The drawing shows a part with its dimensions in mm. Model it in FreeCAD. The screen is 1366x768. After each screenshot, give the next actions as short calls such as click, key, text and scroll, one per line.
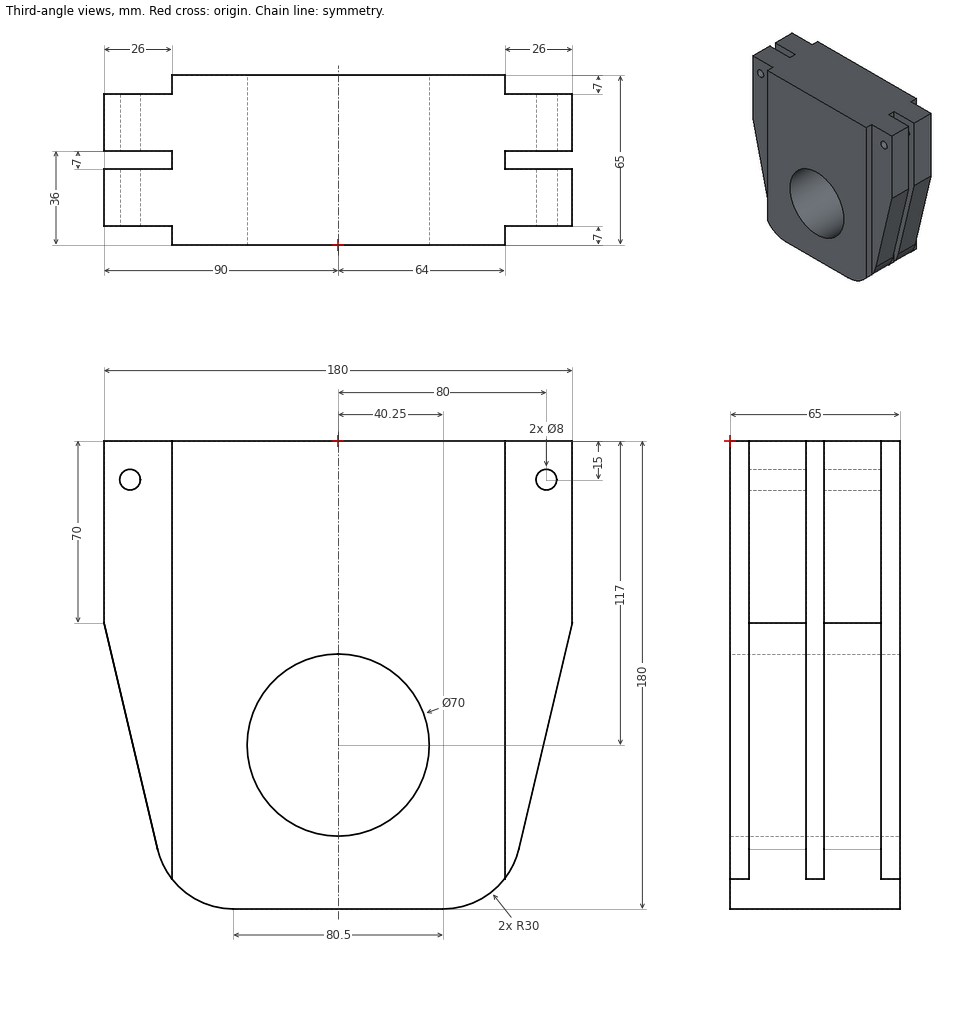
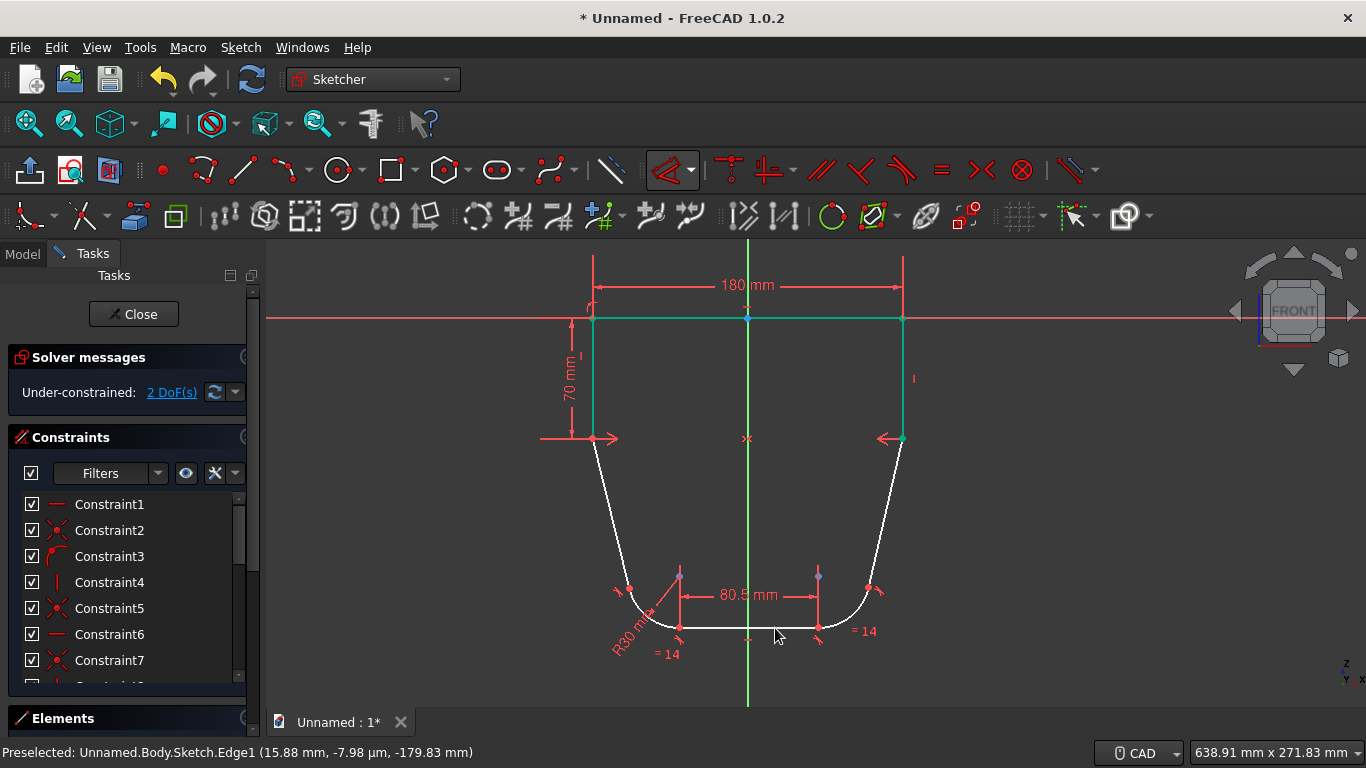
click(818, 628)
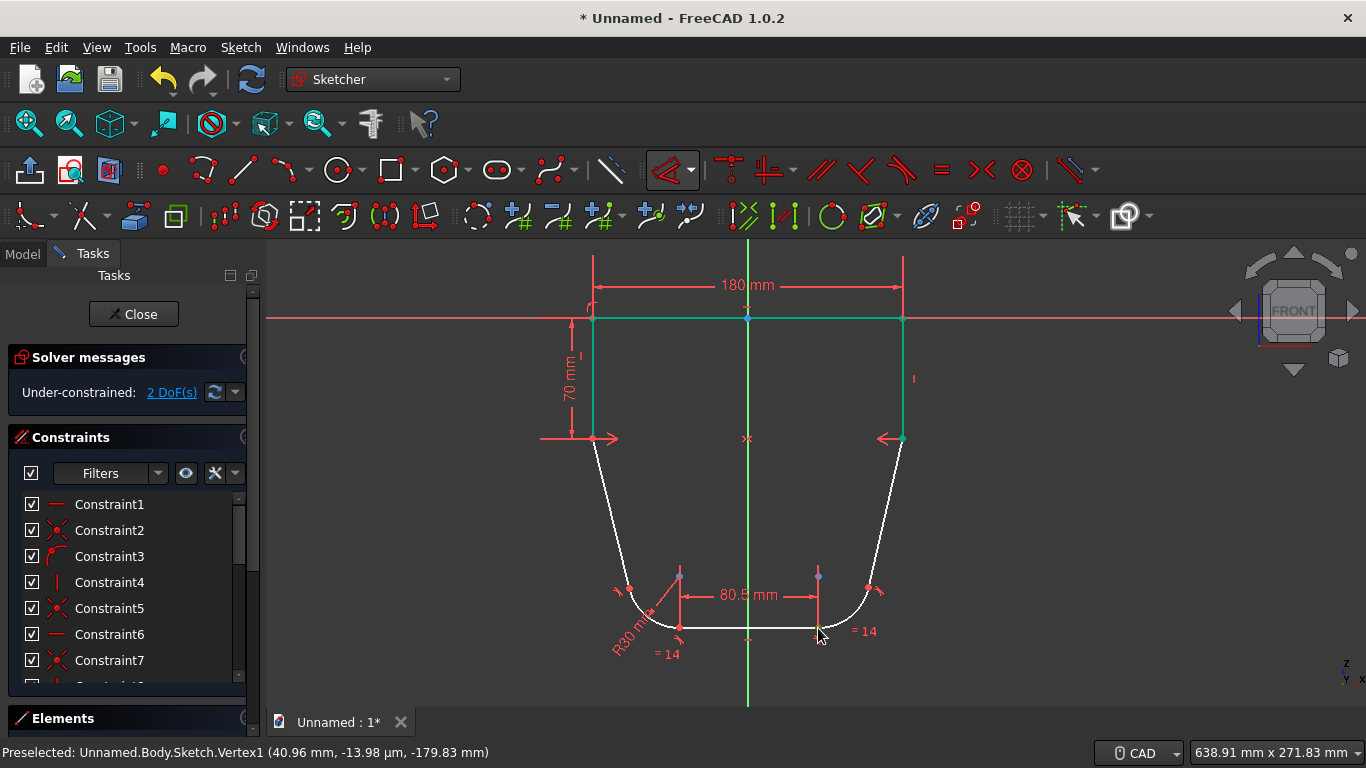
click(694, 170)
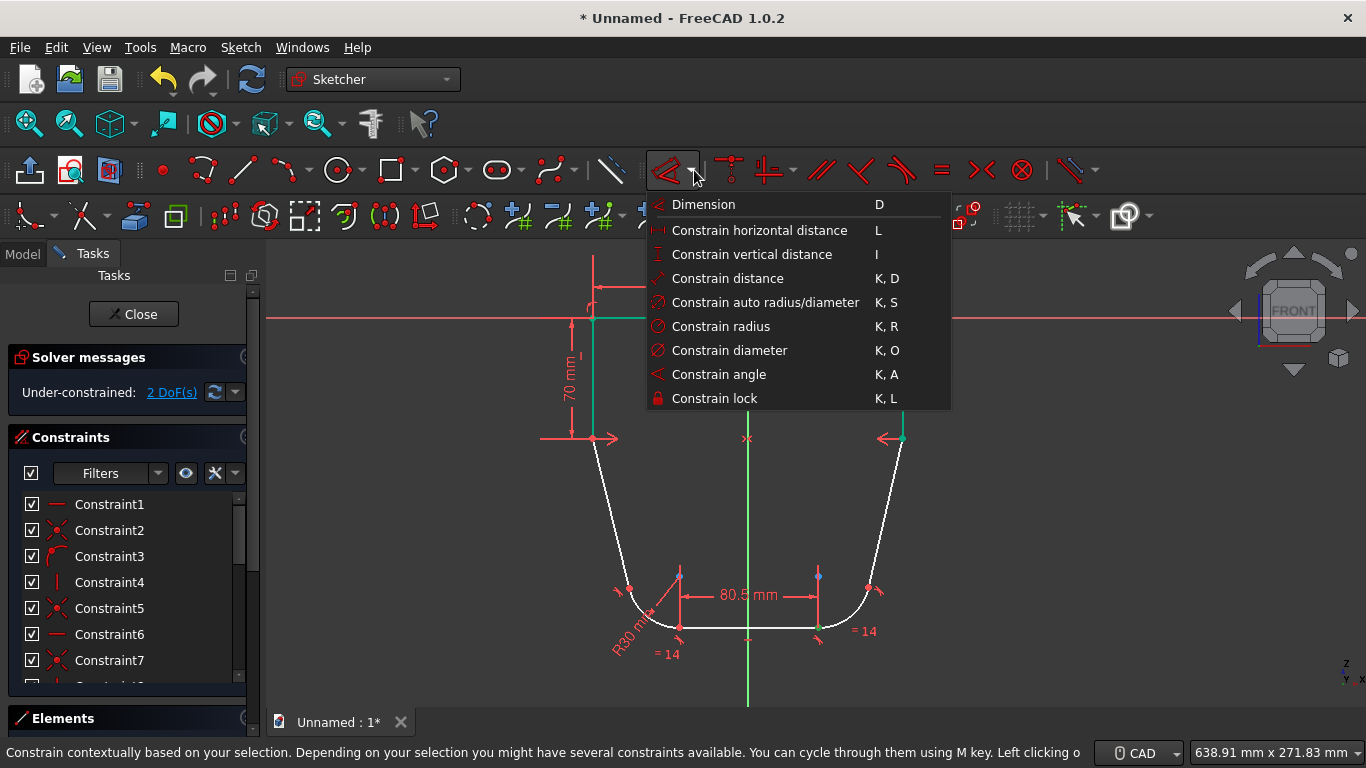
click(799, 254)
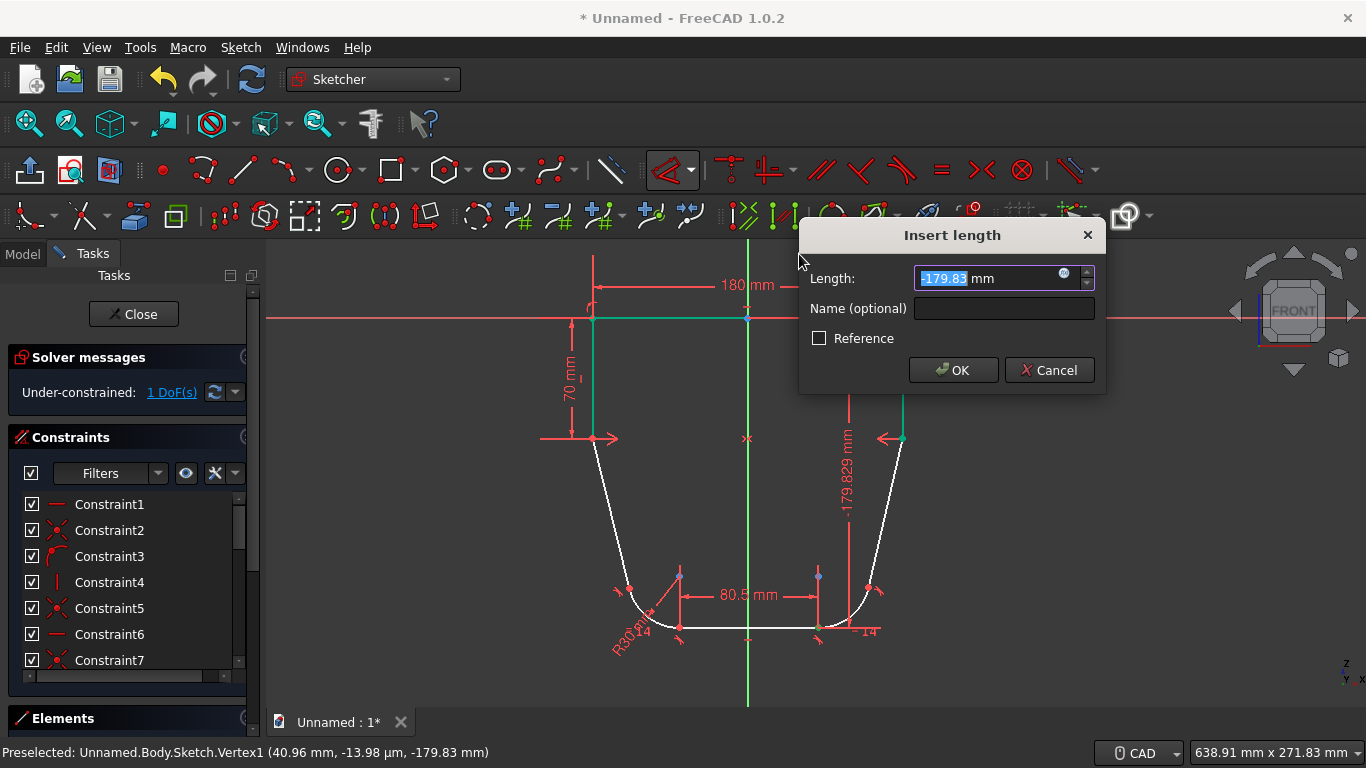
text(-180)
key(Return)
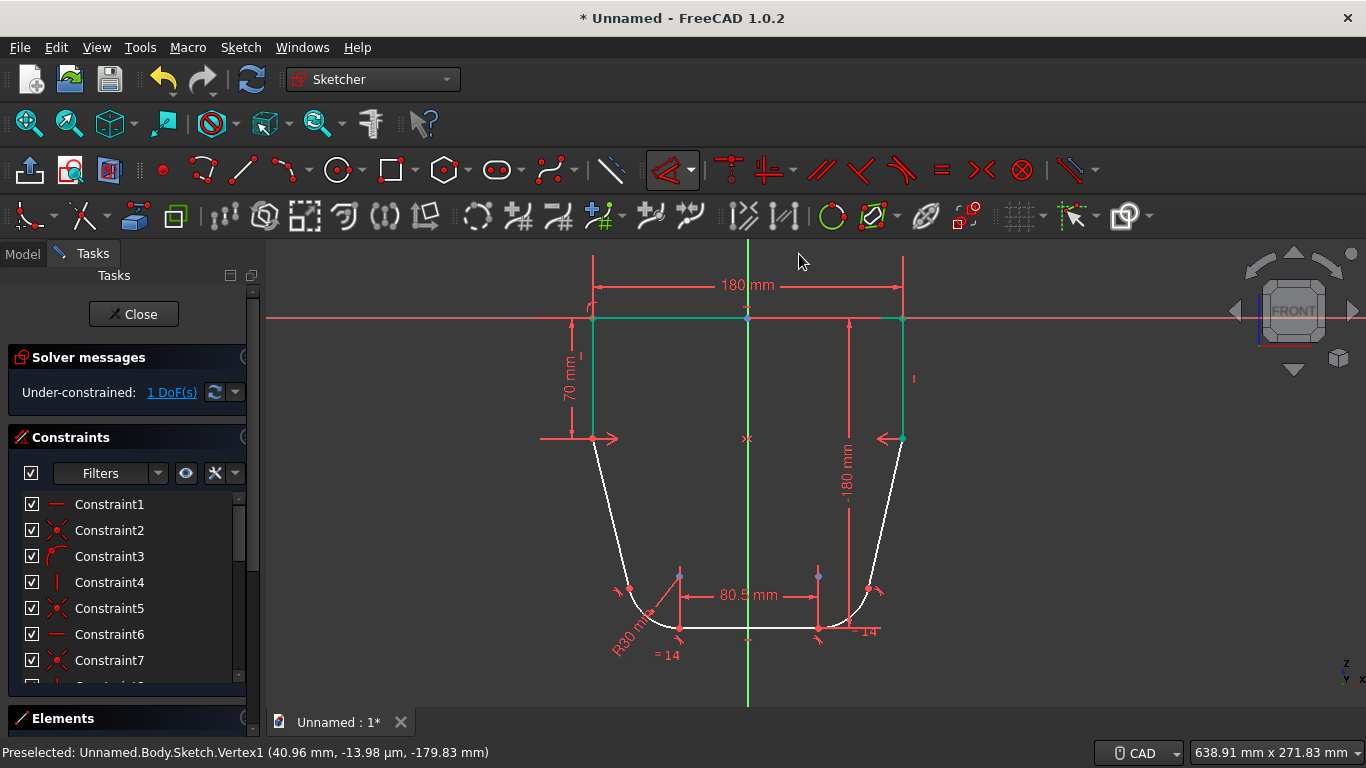
click(818, 628)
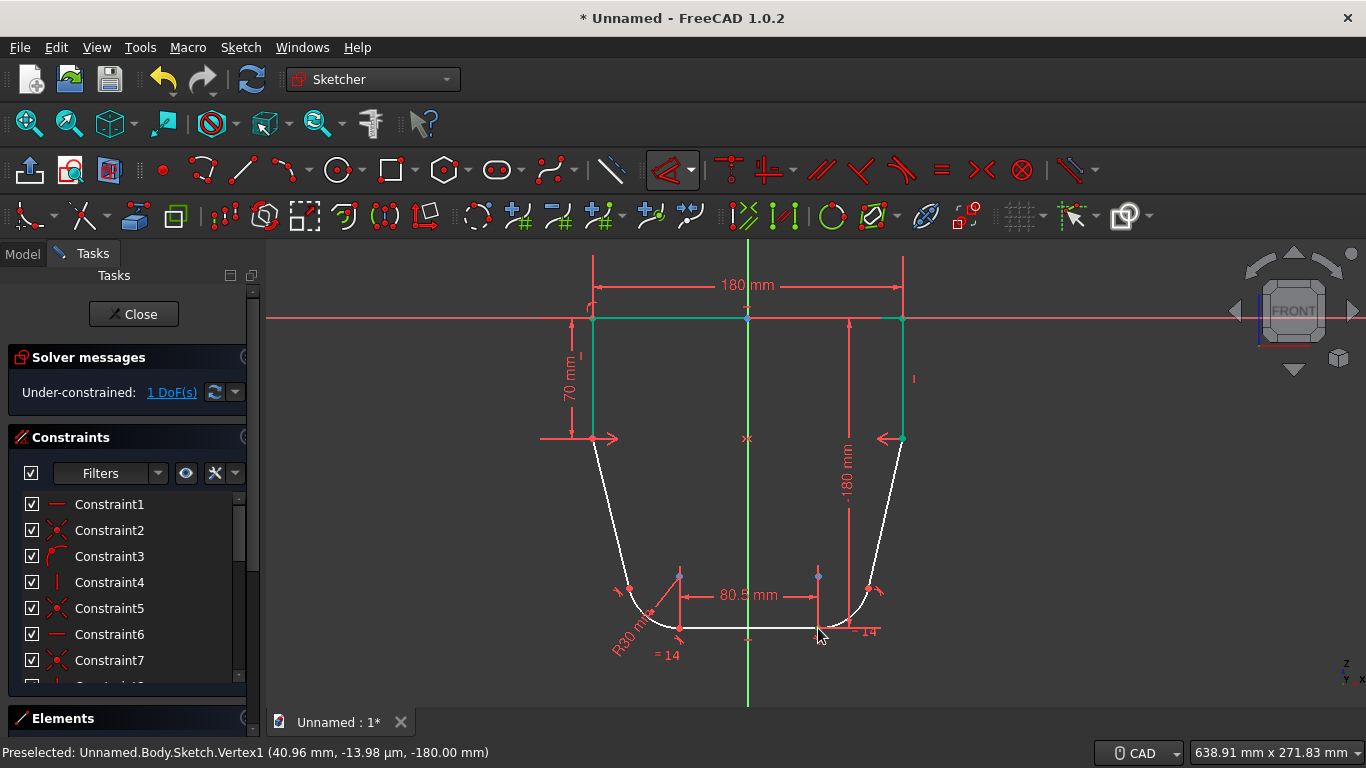
key(l)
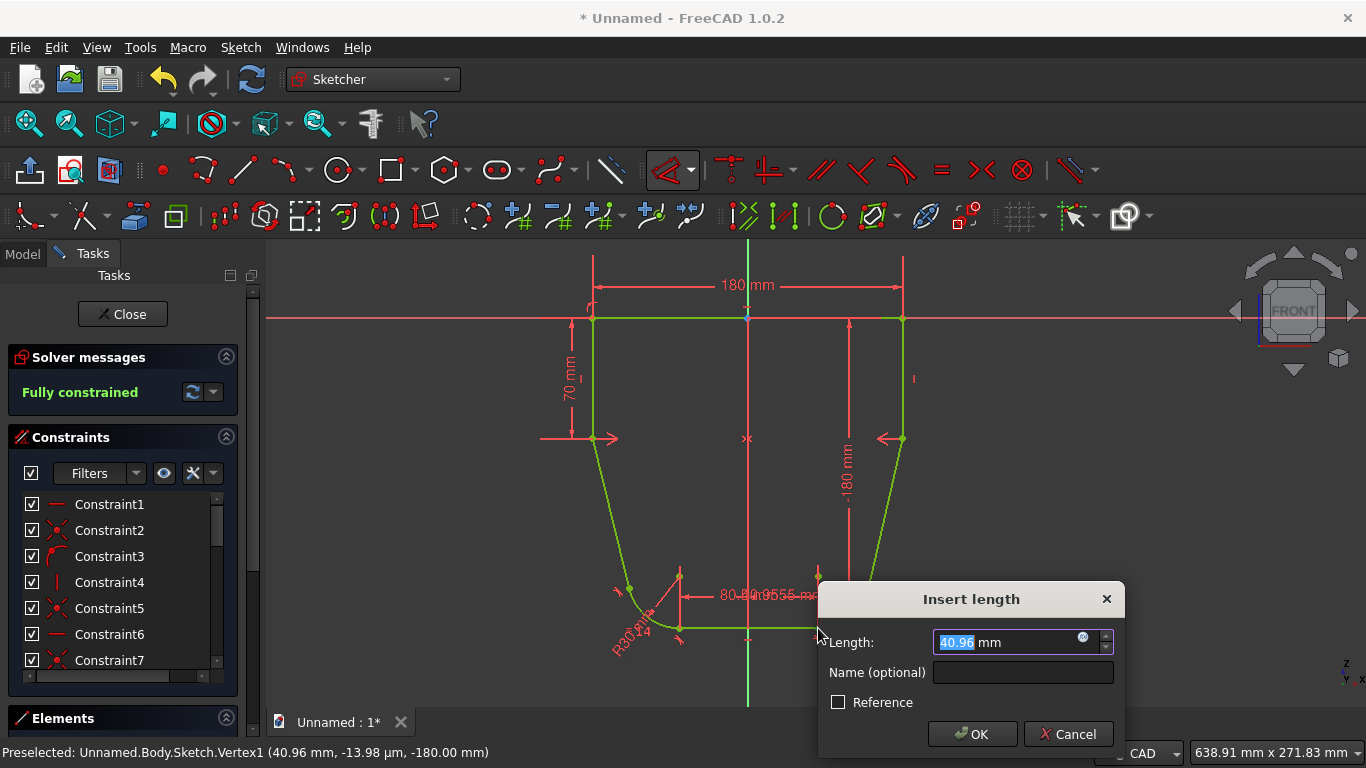
text(40.25)
key(Return)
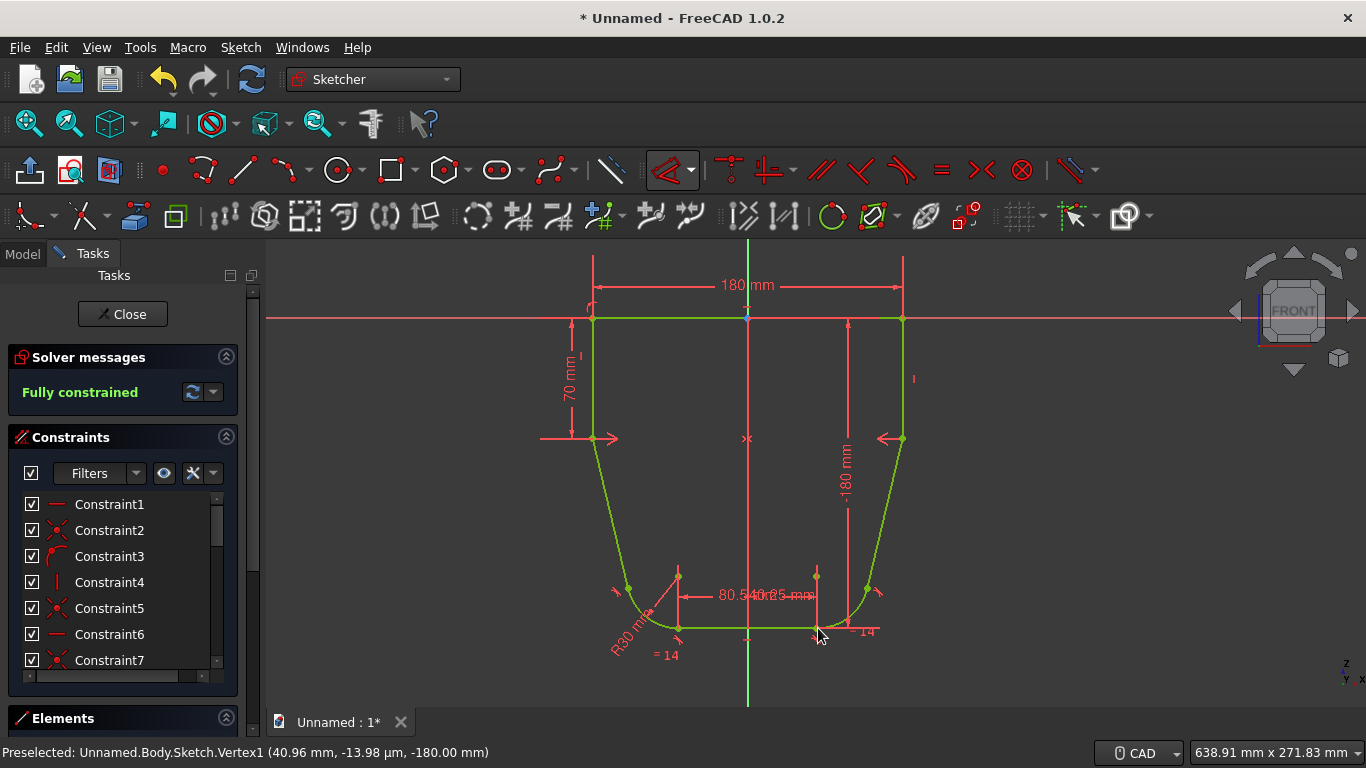
click(123, 314)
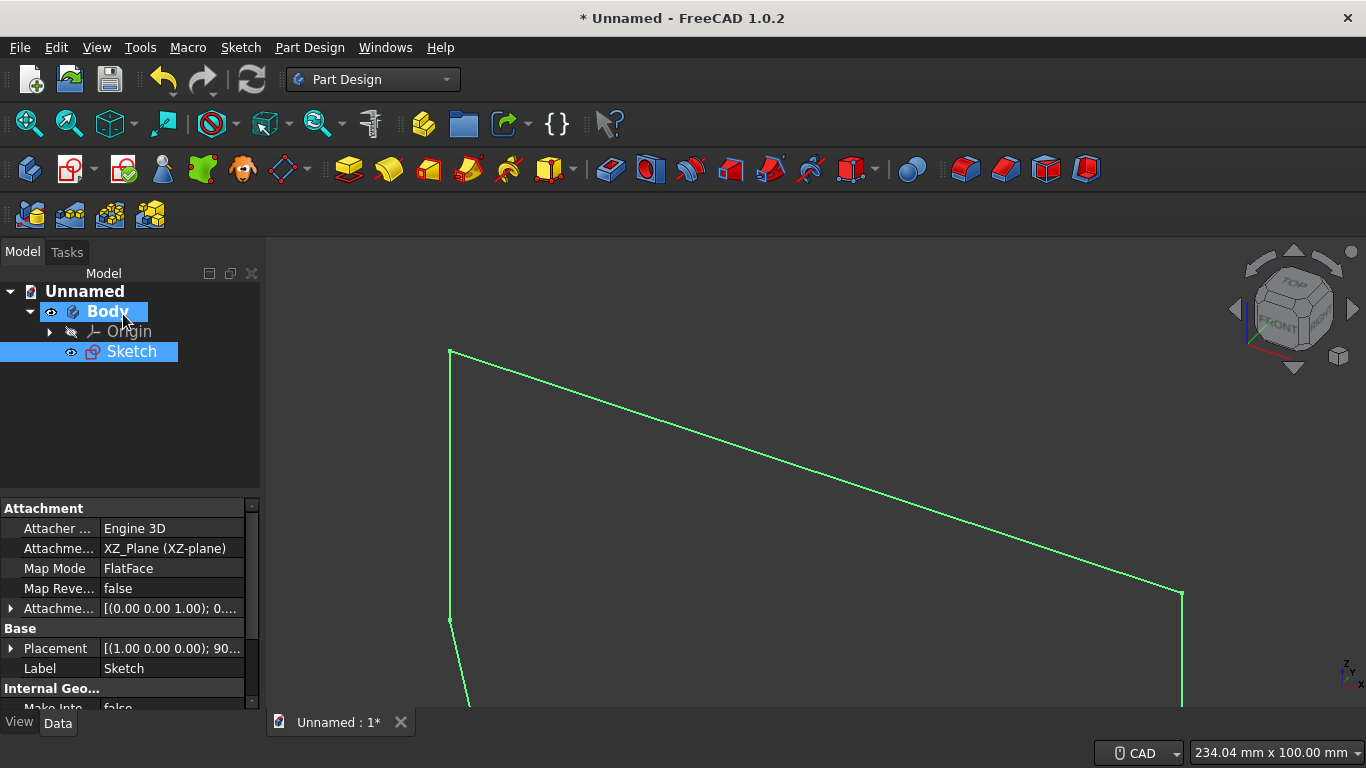
click(350, 170)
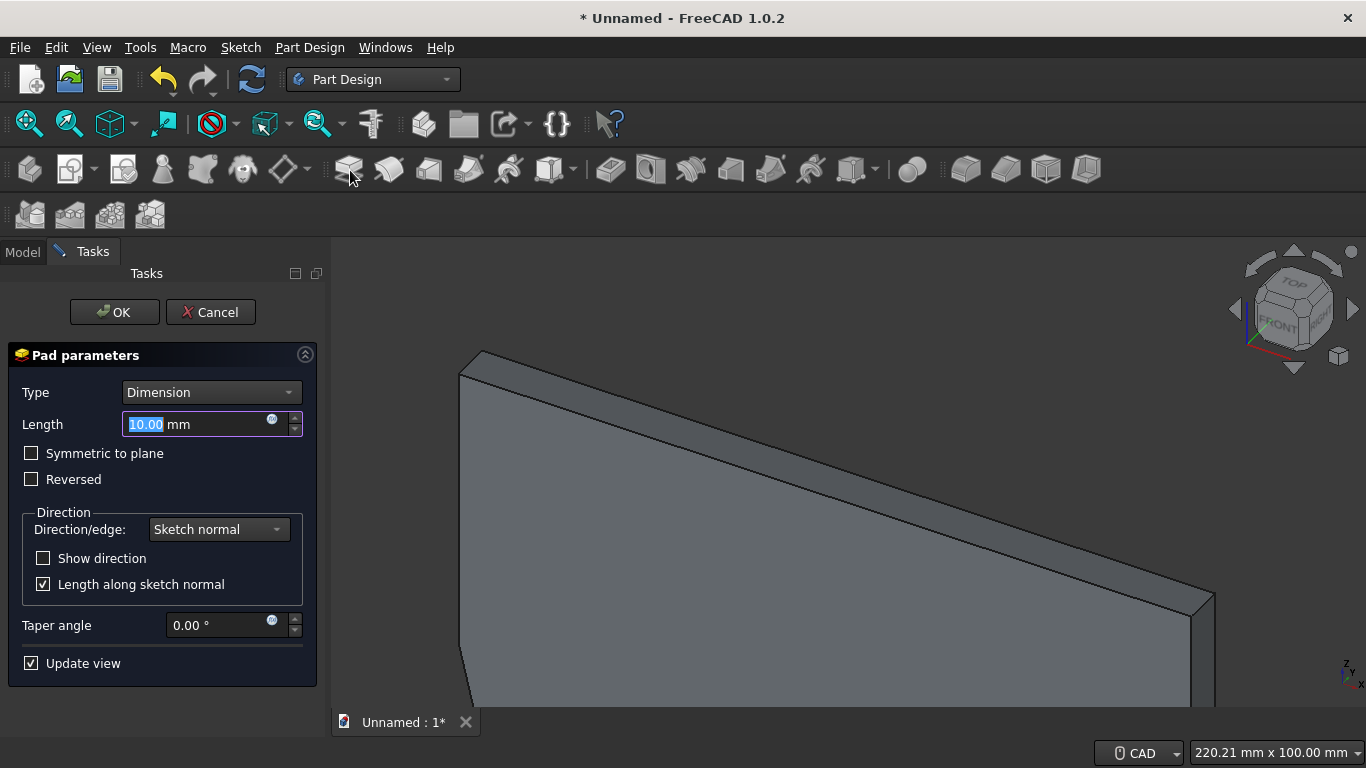
text(65)
key(Tab)